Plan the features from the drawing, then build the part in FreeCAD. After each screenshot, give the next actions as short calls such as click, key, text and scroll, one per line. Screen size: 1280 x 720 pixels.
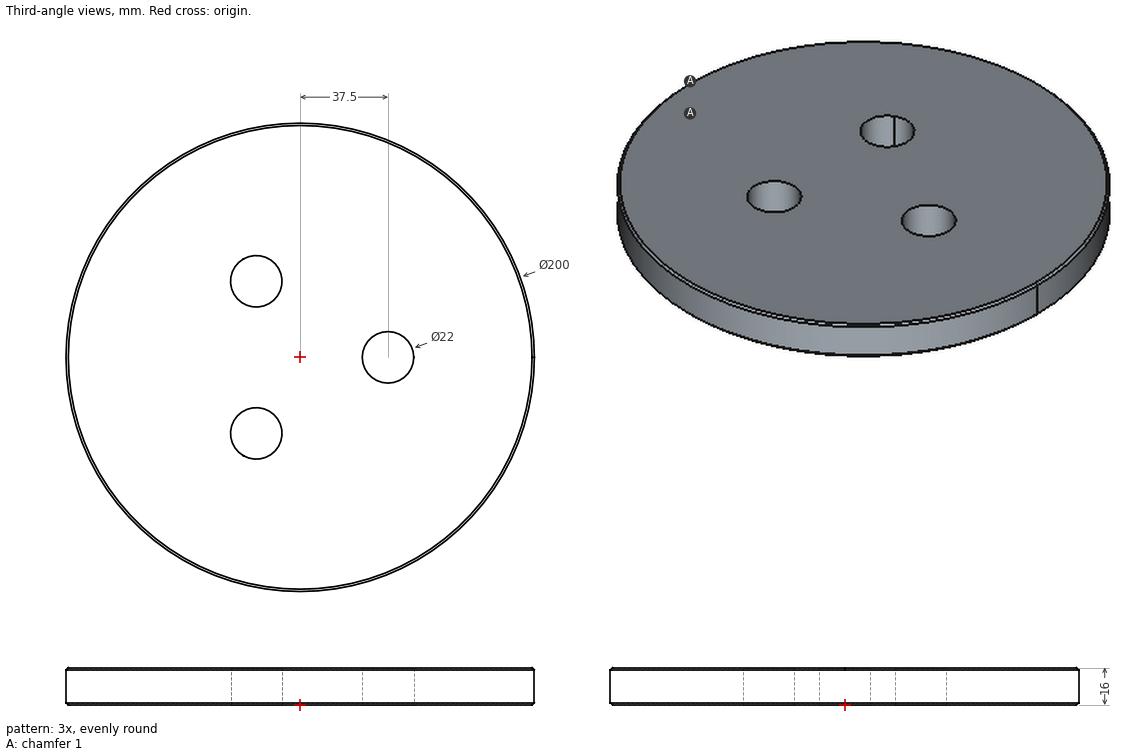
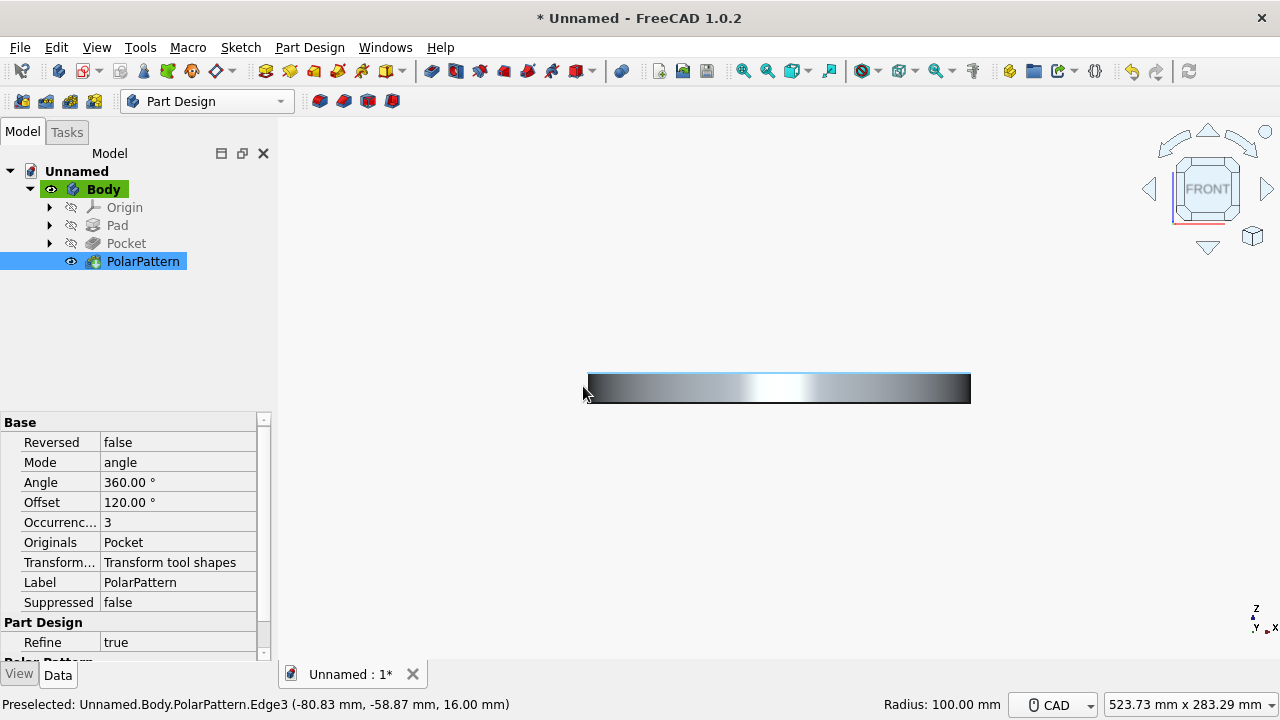
key(v)
key(f)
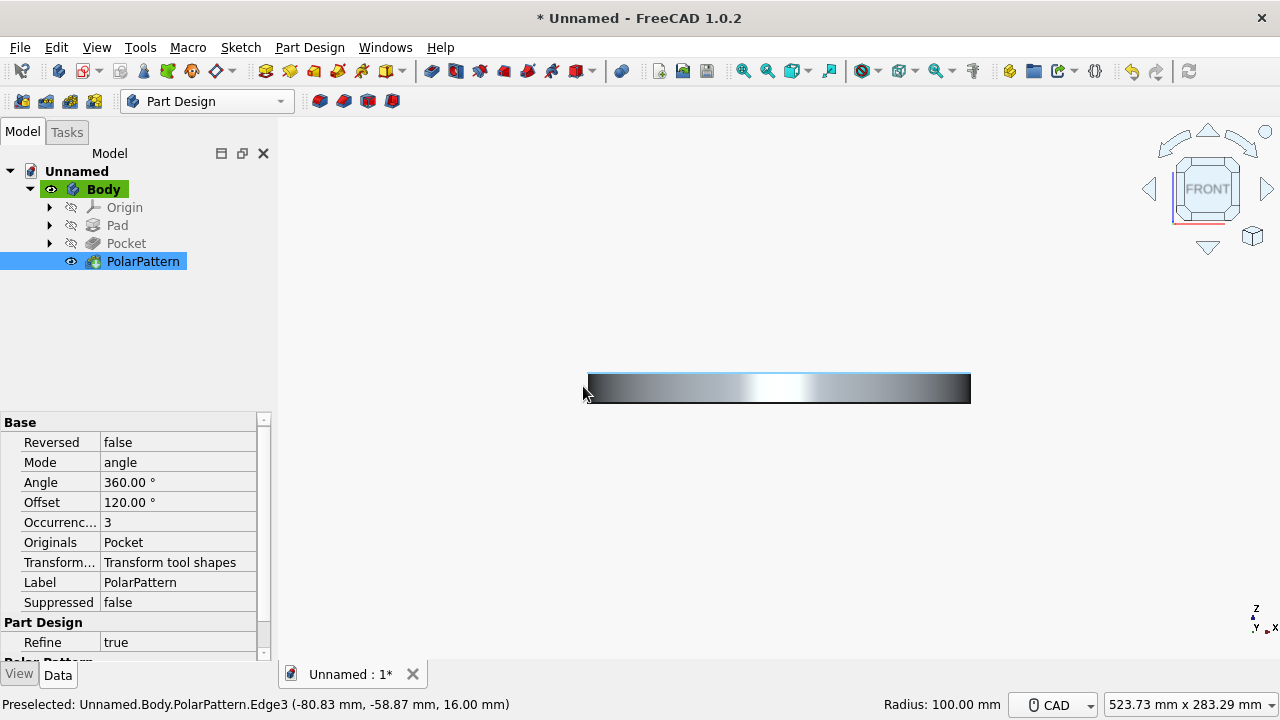
click(624, 402, ctrl)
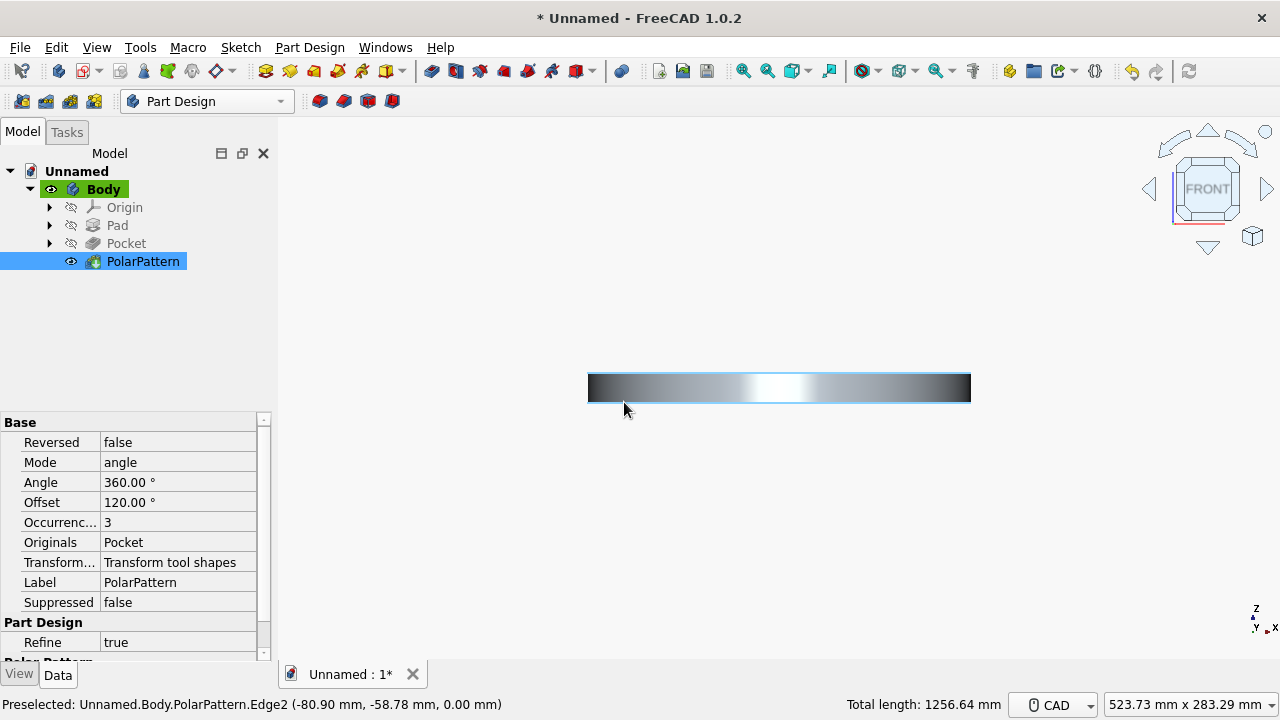
click(344, 102)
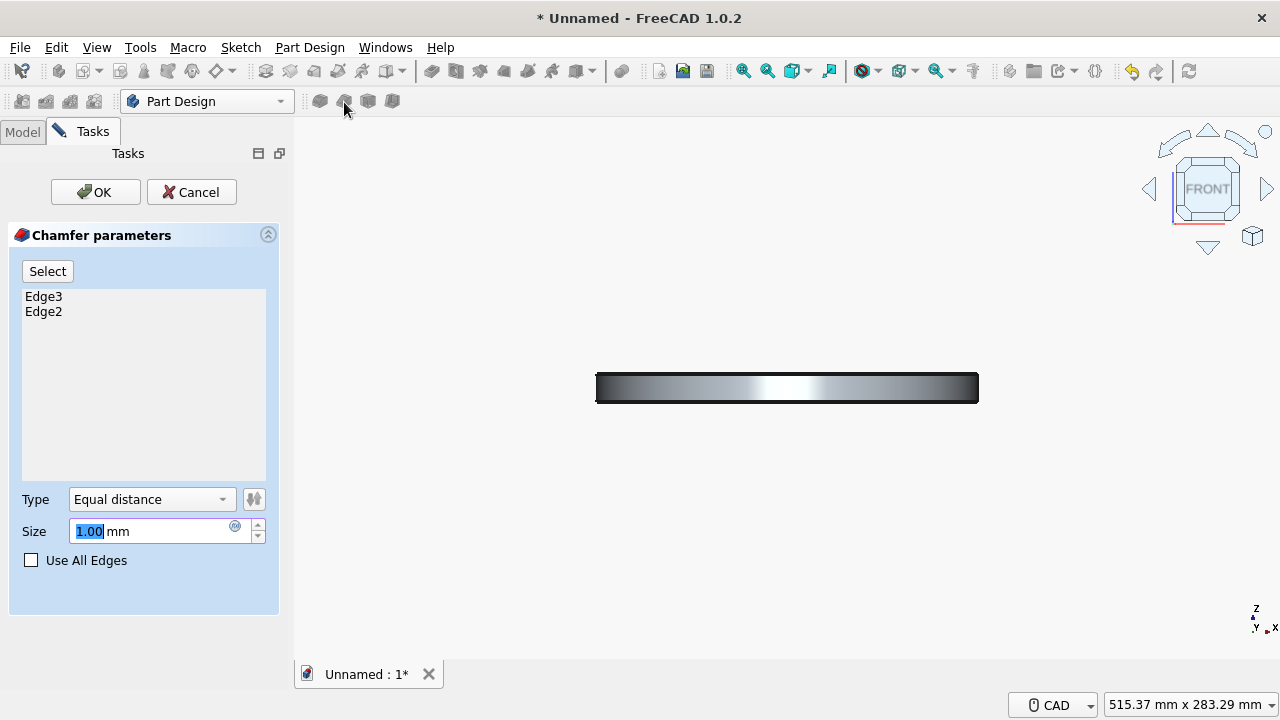
text(1)
key(Tab)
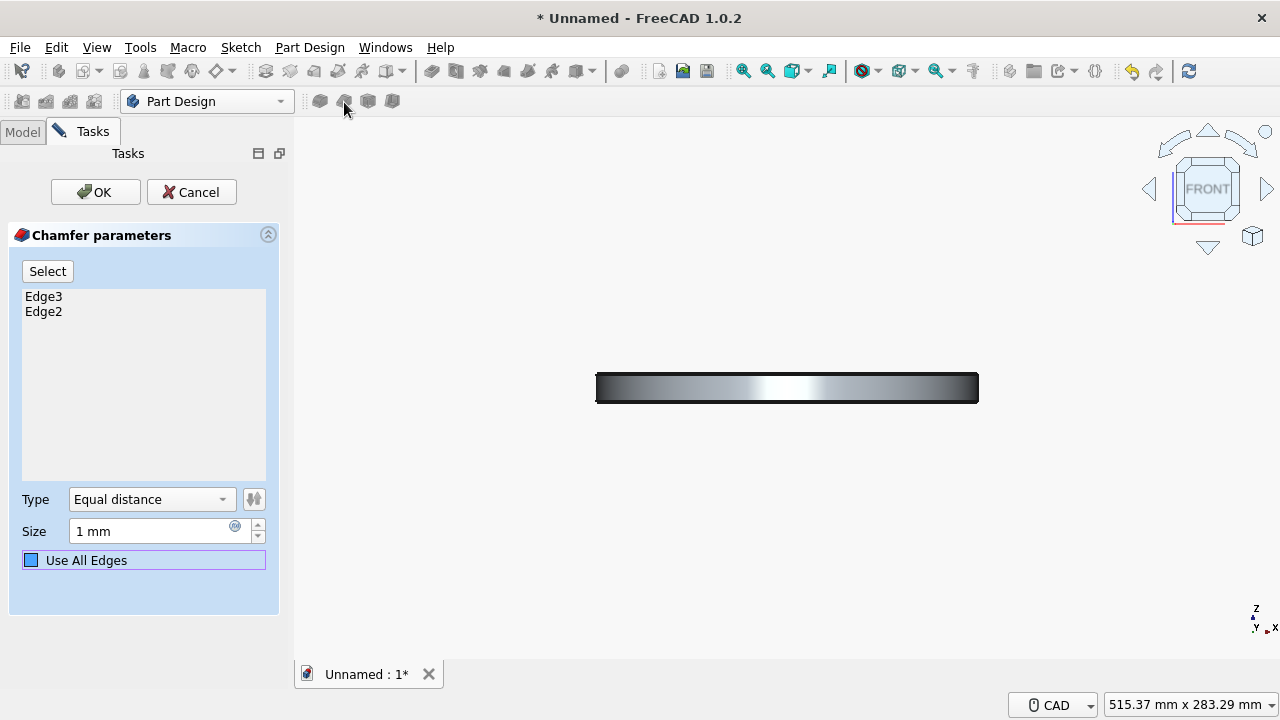
click(96, 192)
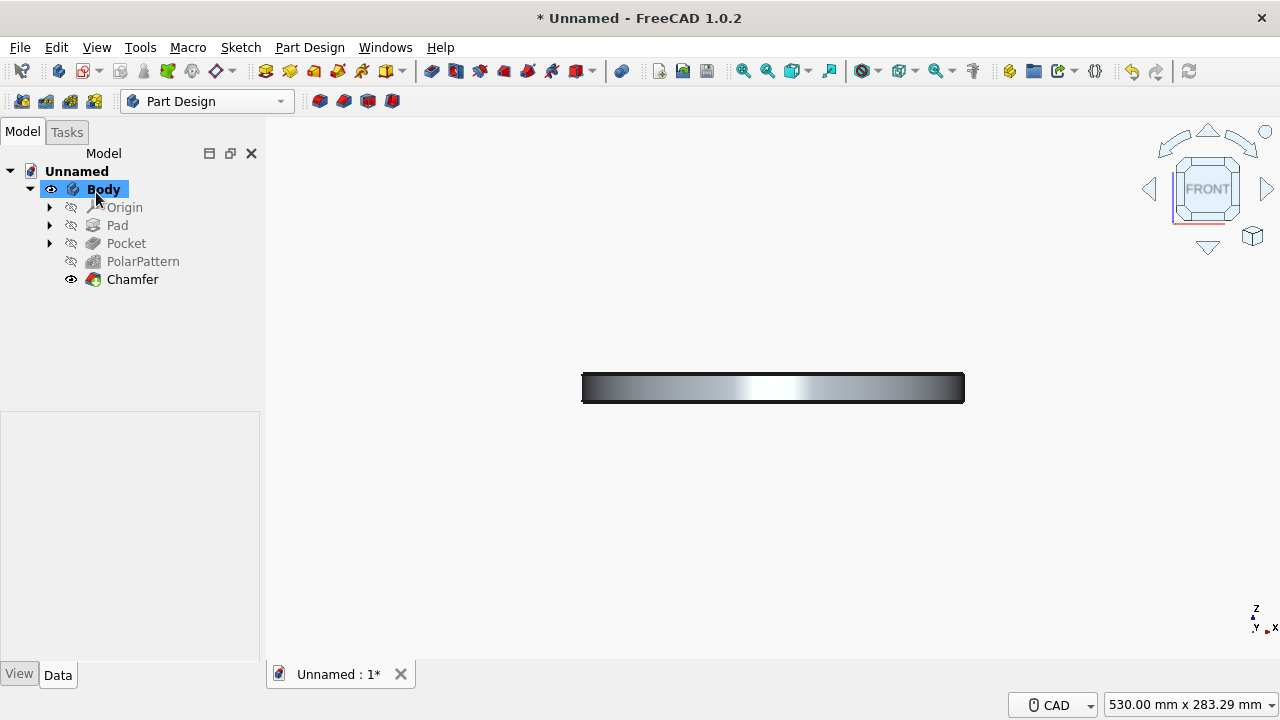
key(0)